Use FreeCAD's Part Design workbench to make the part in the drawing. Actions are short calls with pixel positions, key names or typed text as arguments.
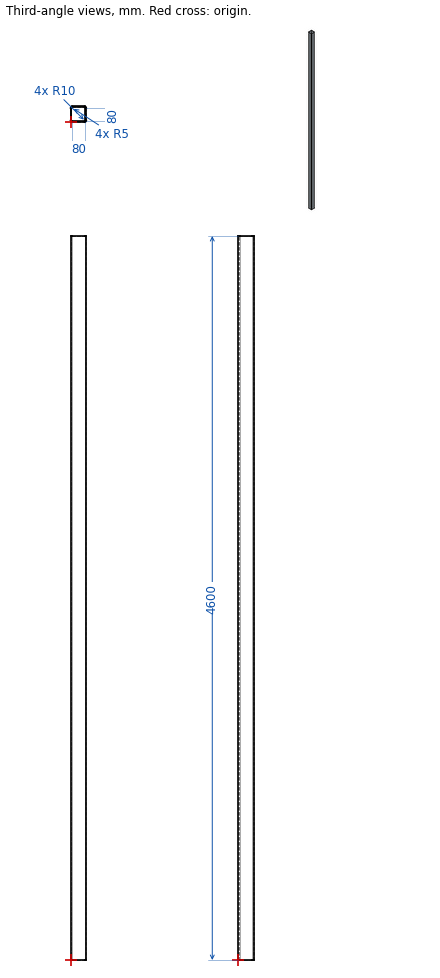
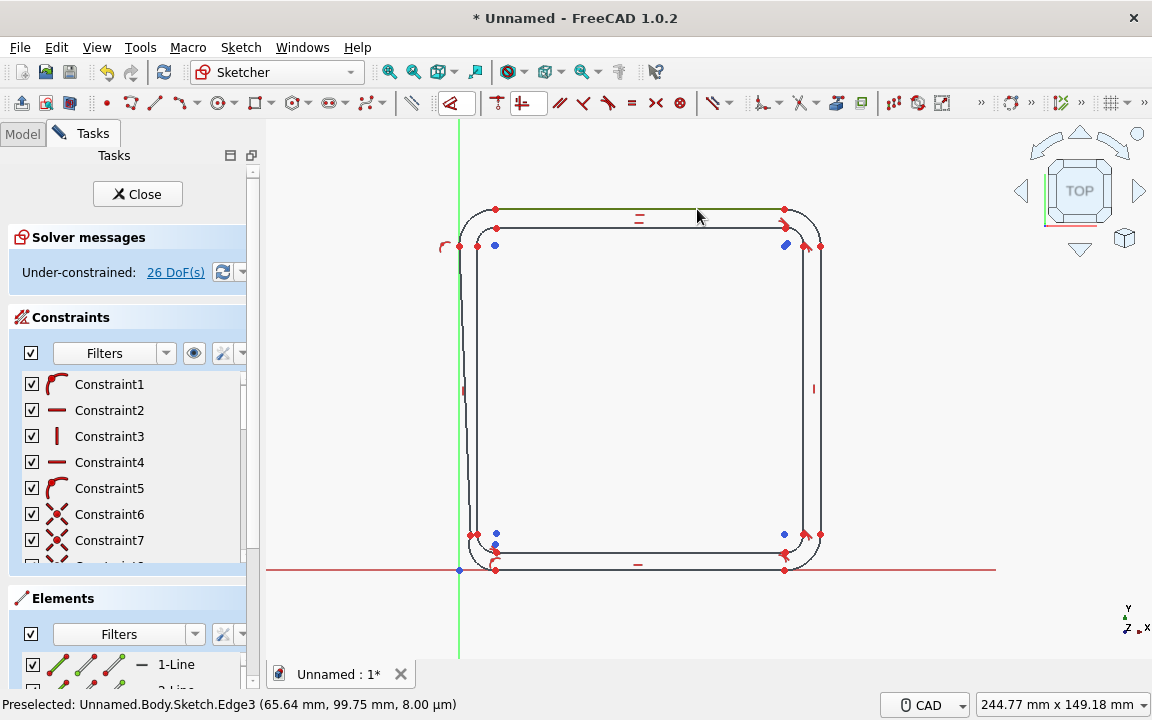
click(479, 213)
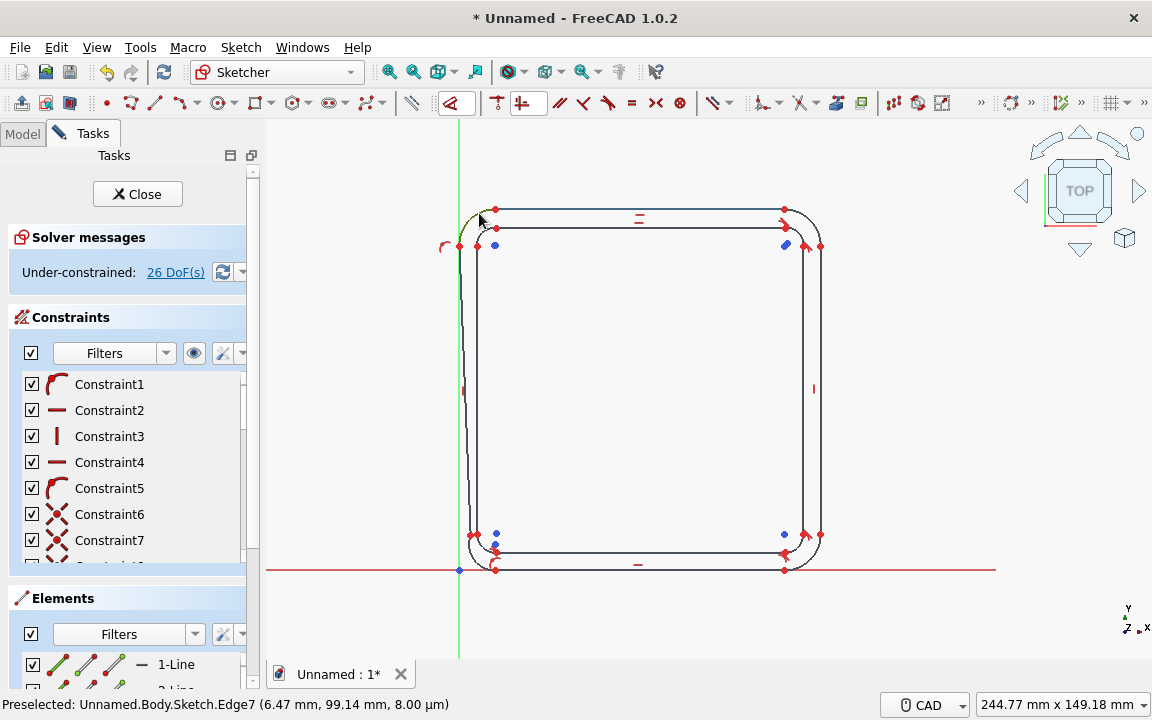
key(t)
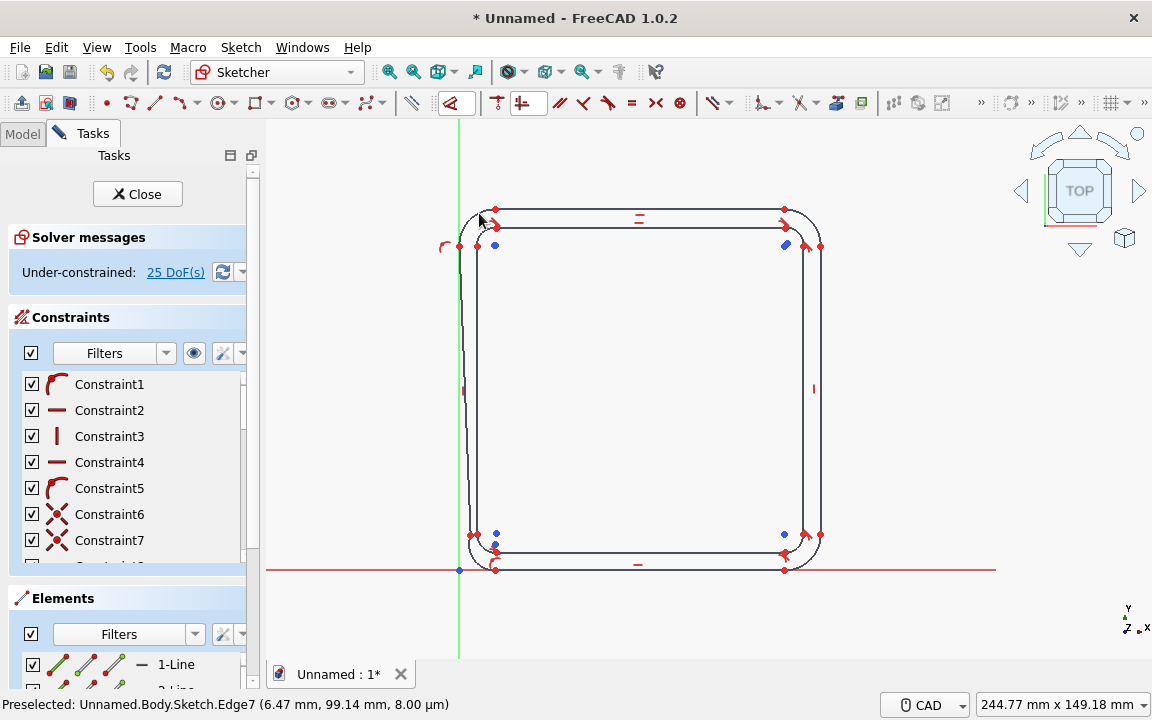
click(463, 333)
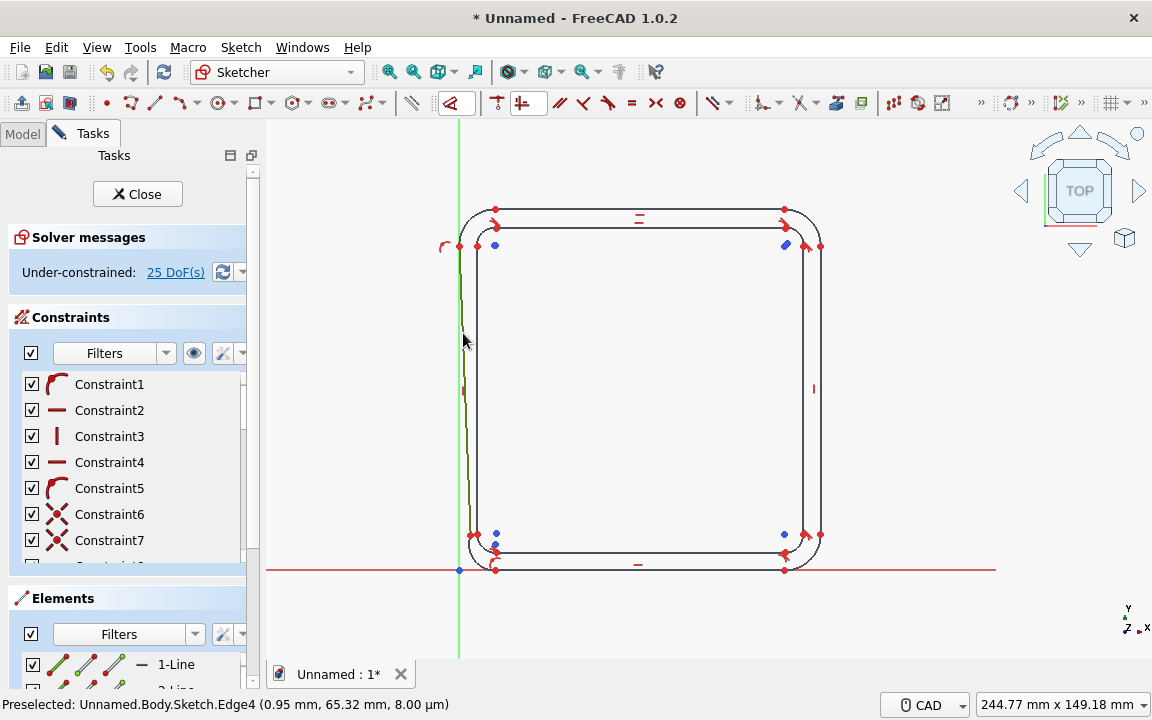
click(479, 213)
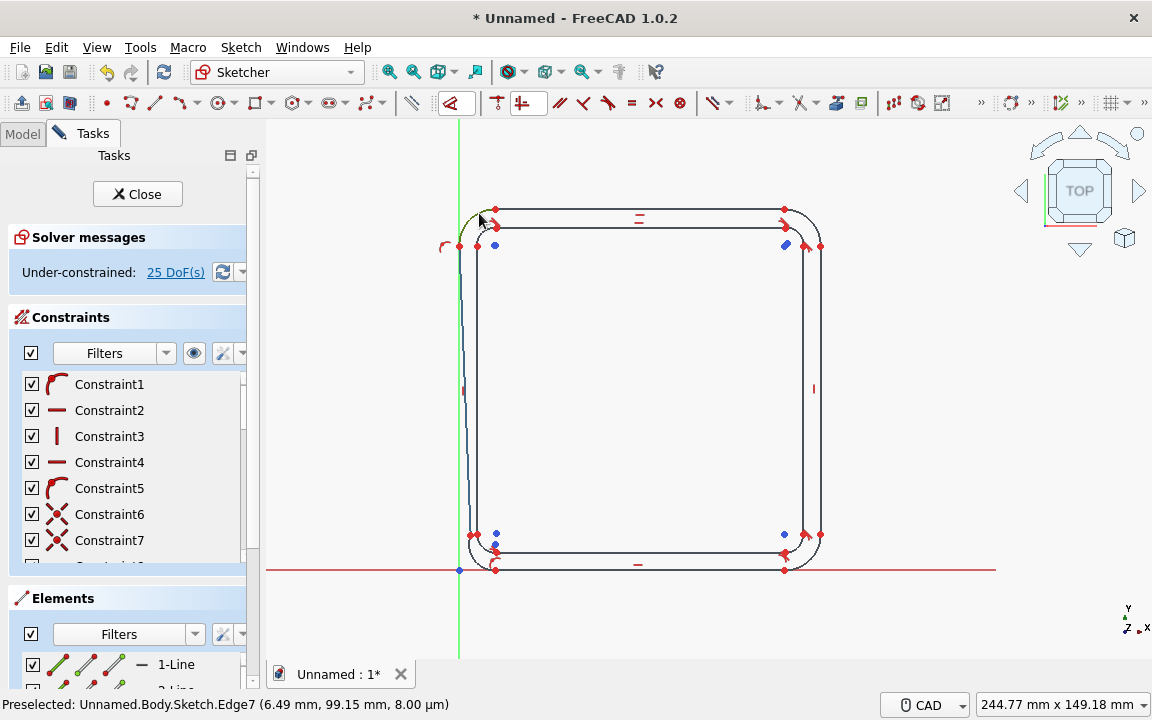
click(608, 104)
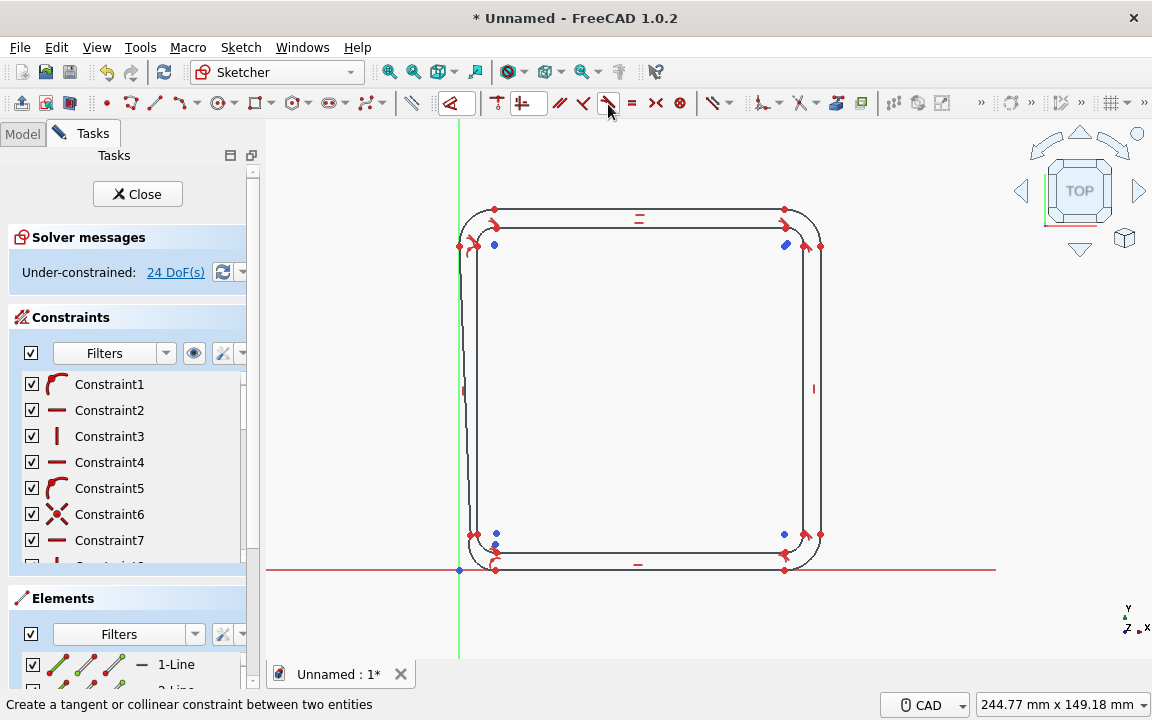
click(463, 333)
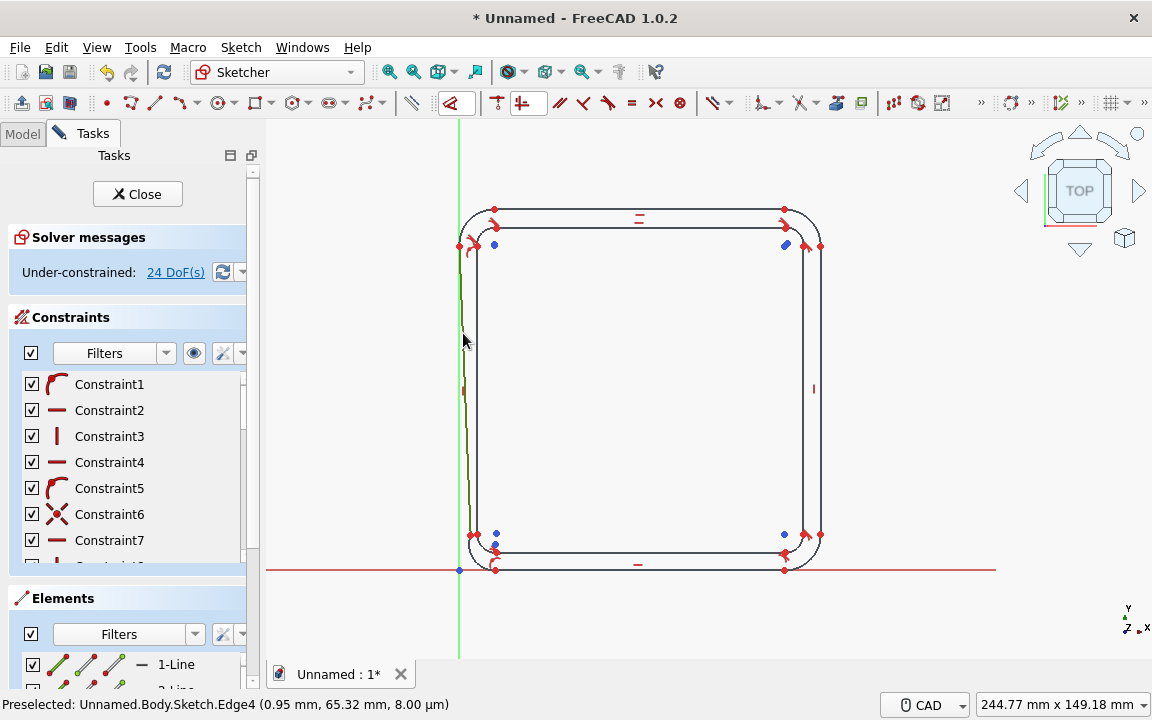
scroll(470, 550, up, 2)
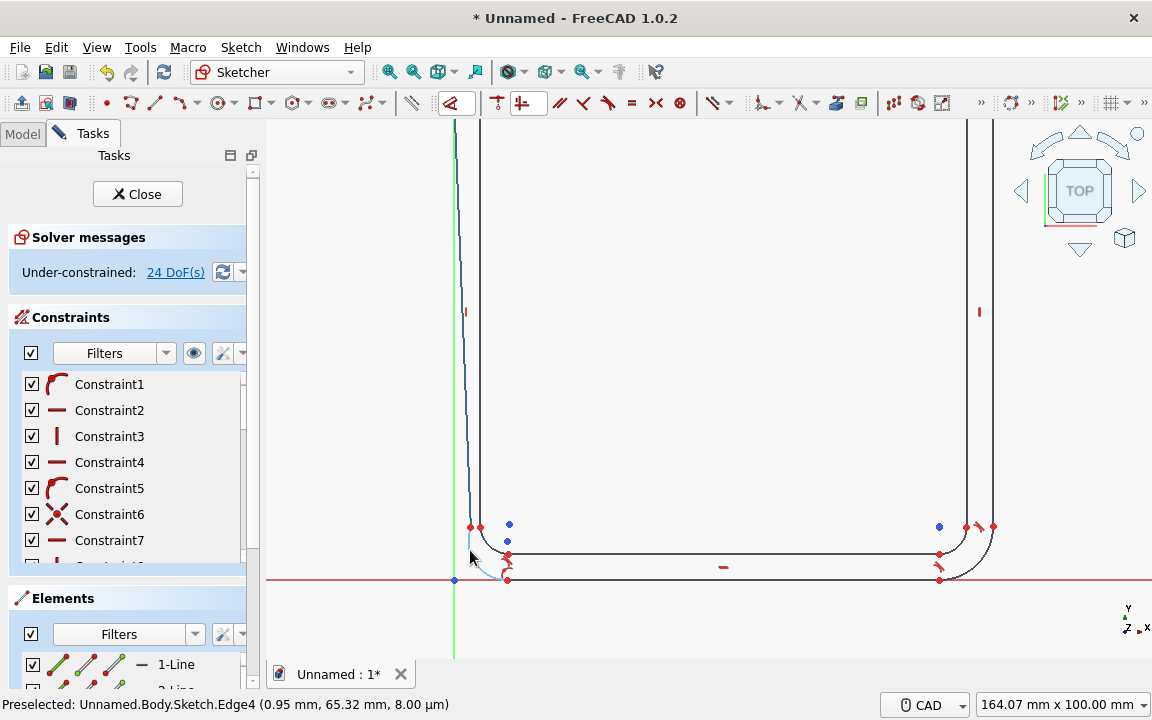
click(469, 550)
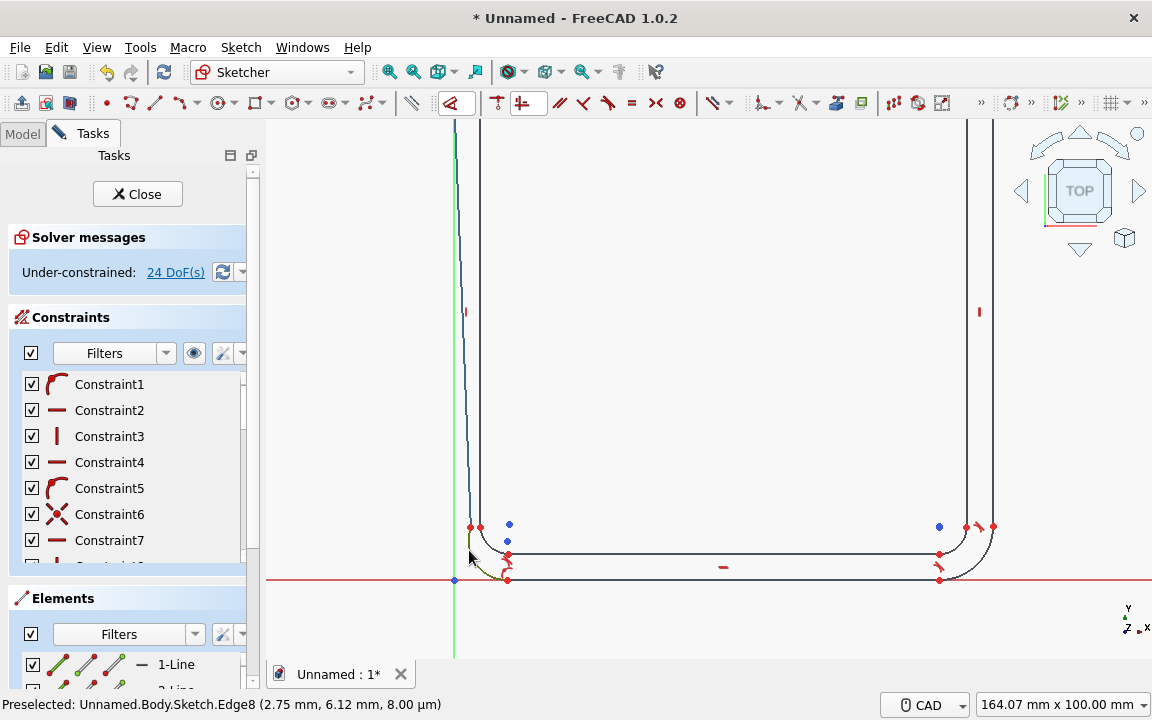
click(608, 104)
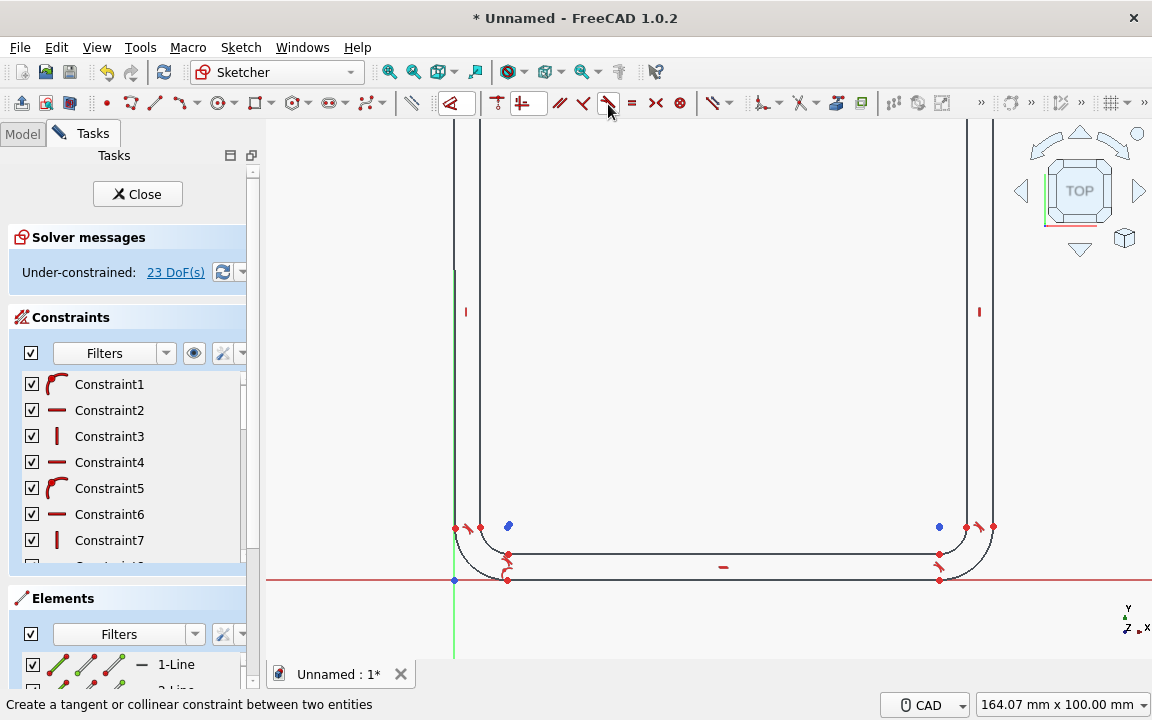
scroll(471, 549, down, 2)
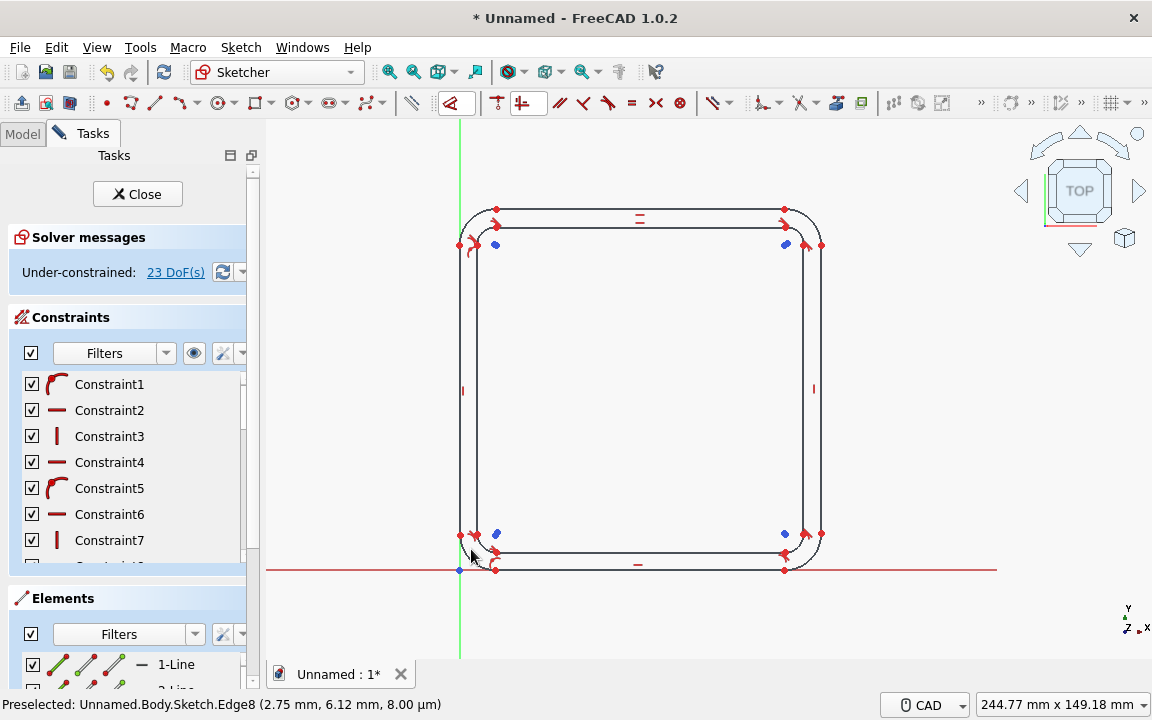
click(583, 228)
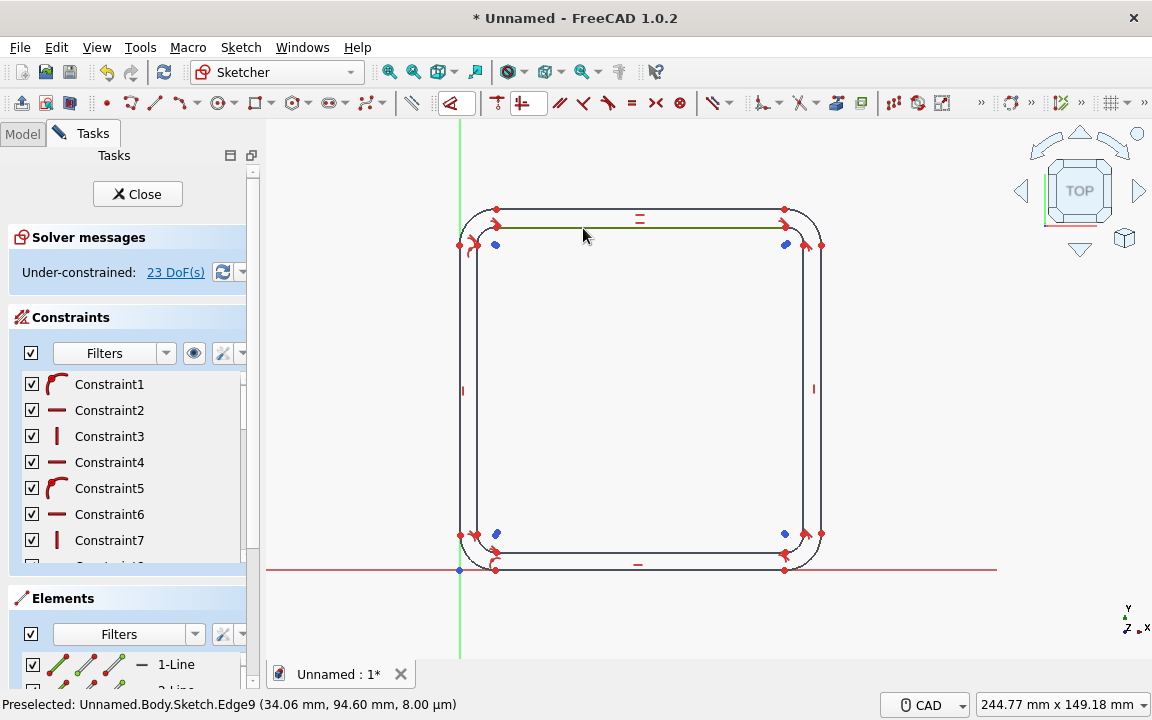
click(799, 232)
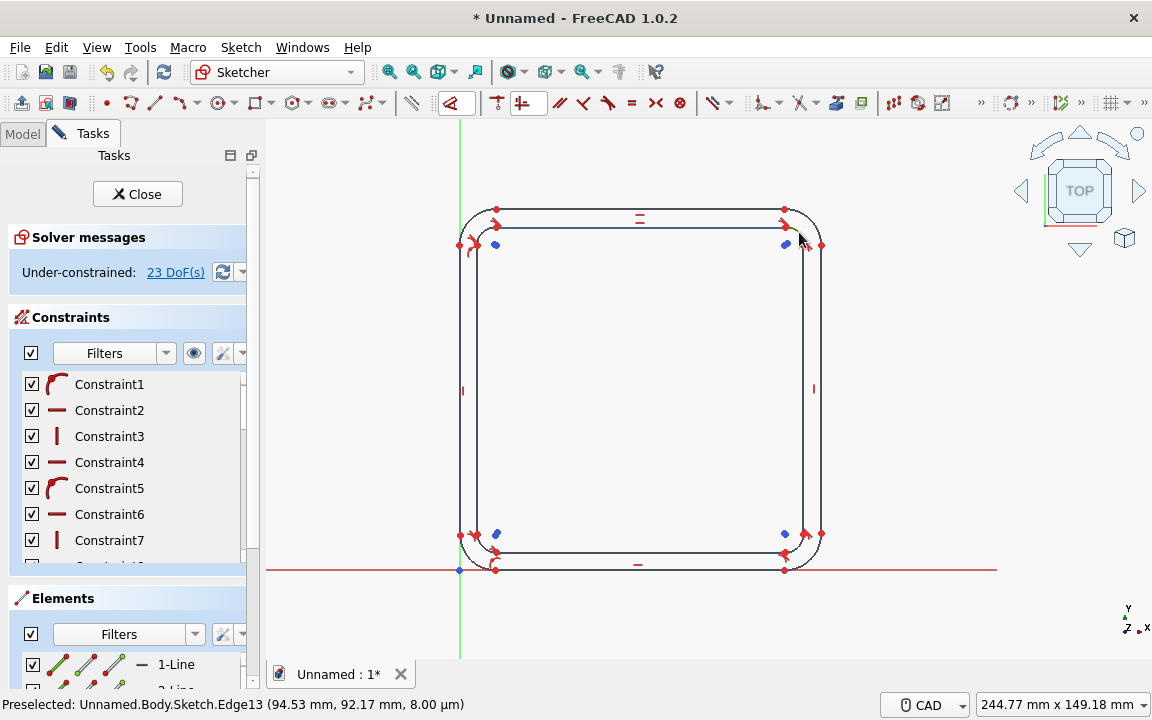
click(608, 104)